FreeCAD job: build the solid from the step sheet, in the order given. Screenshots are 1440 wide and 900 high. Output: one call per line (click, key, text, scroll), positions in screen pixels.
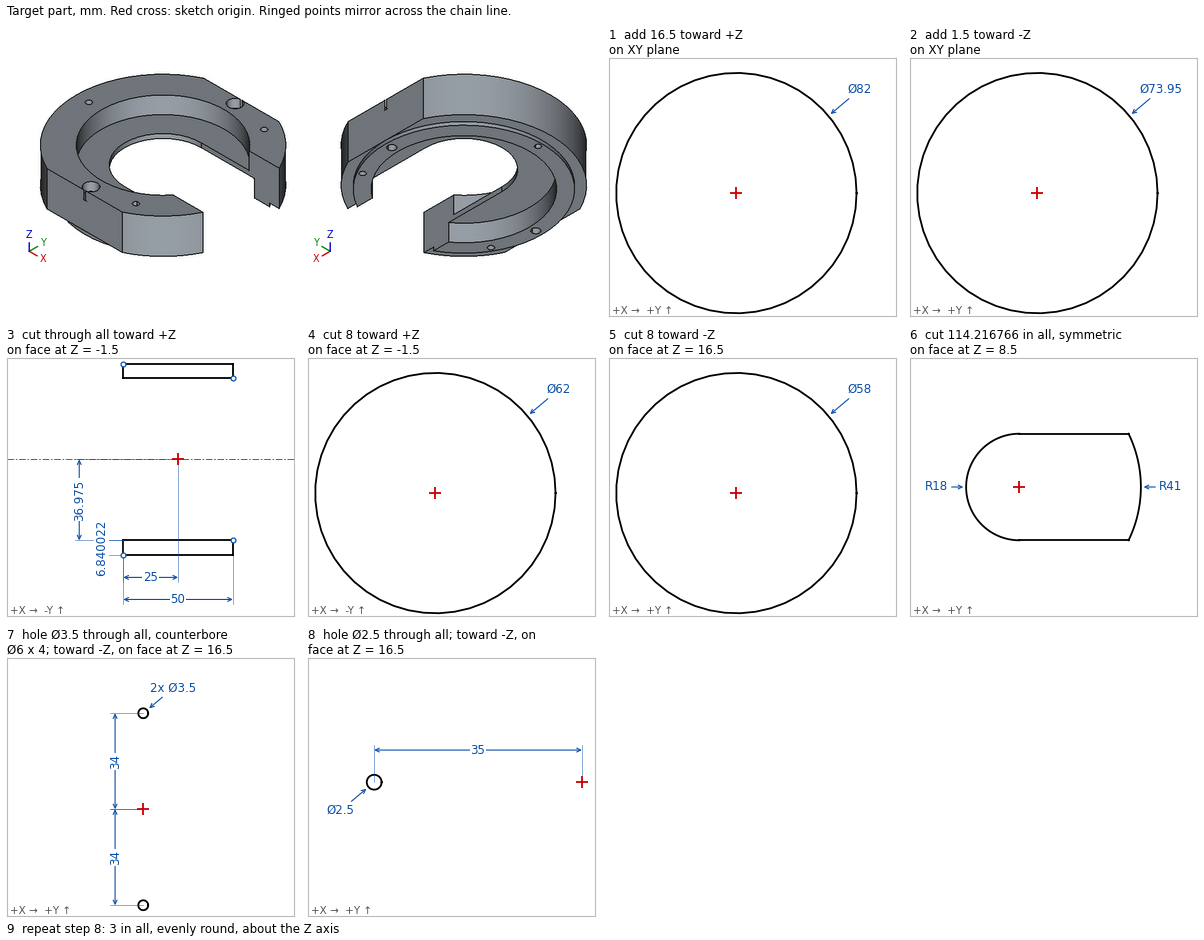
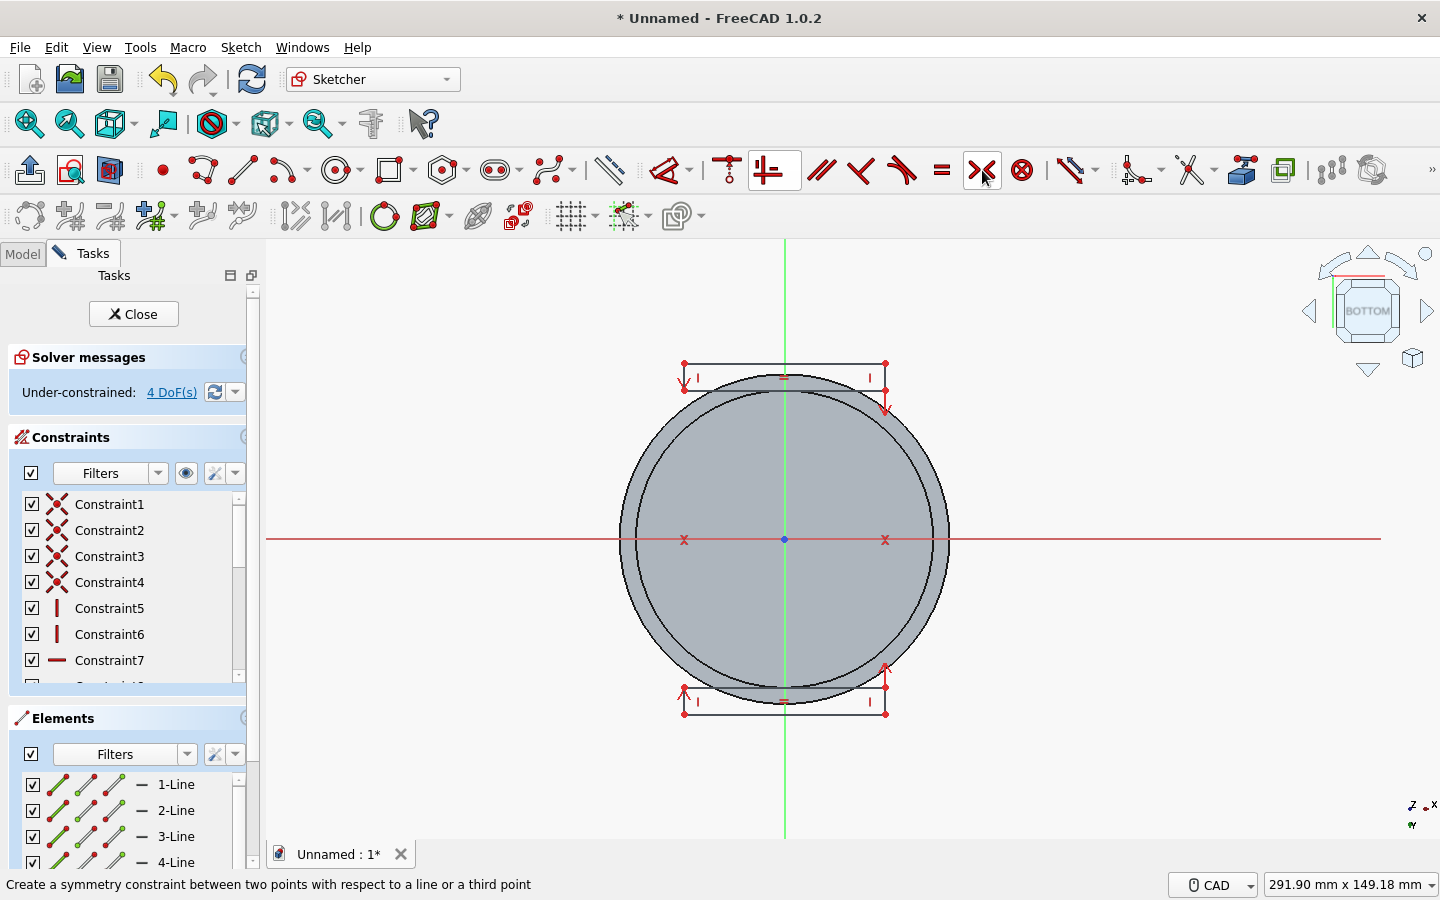
click(664, 170)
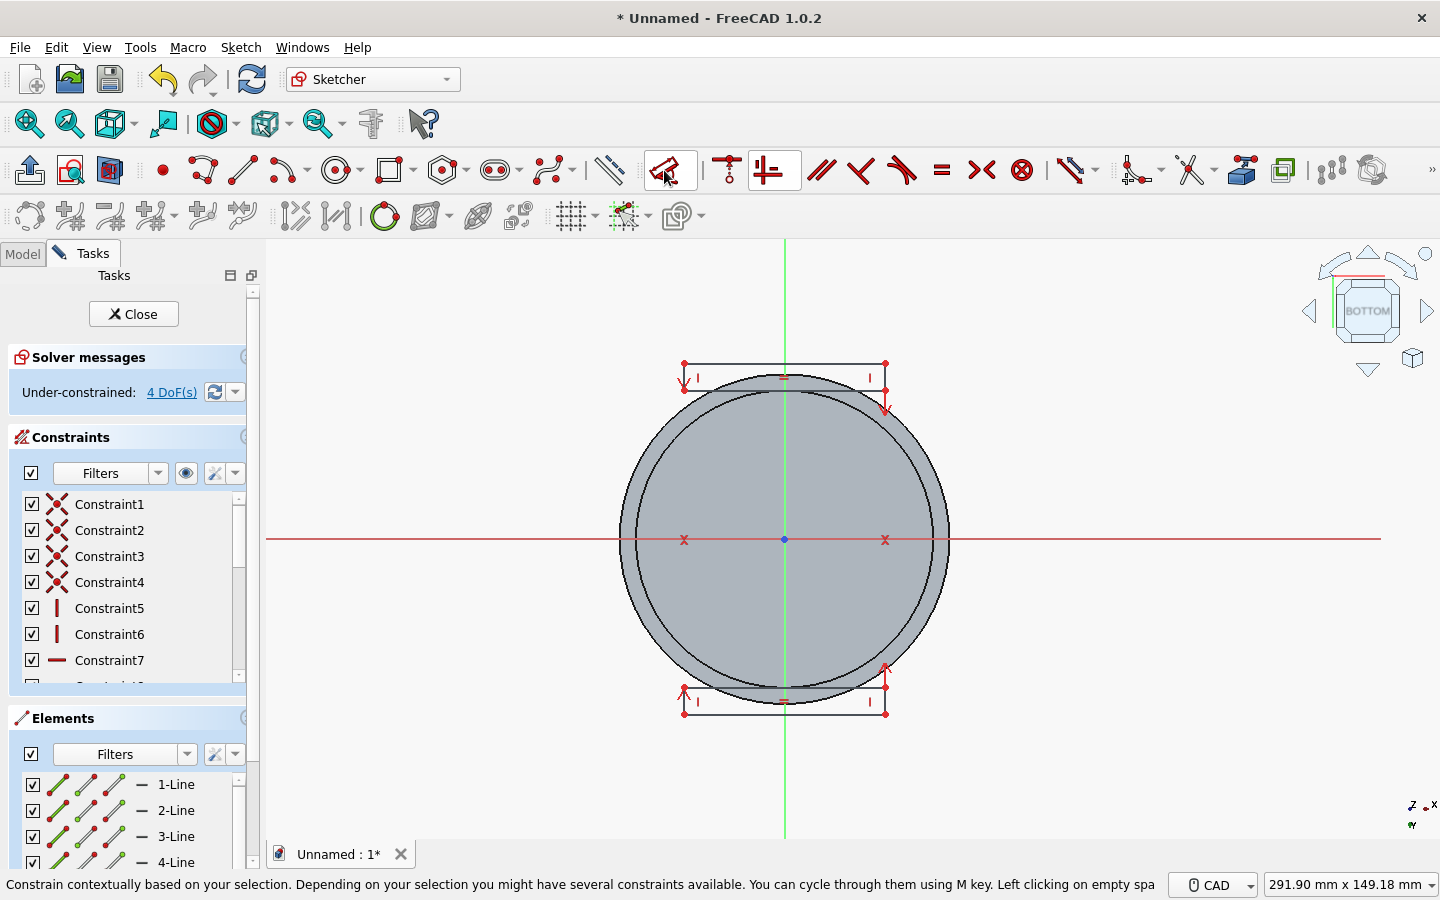
click(744, 715)
click(738, 749)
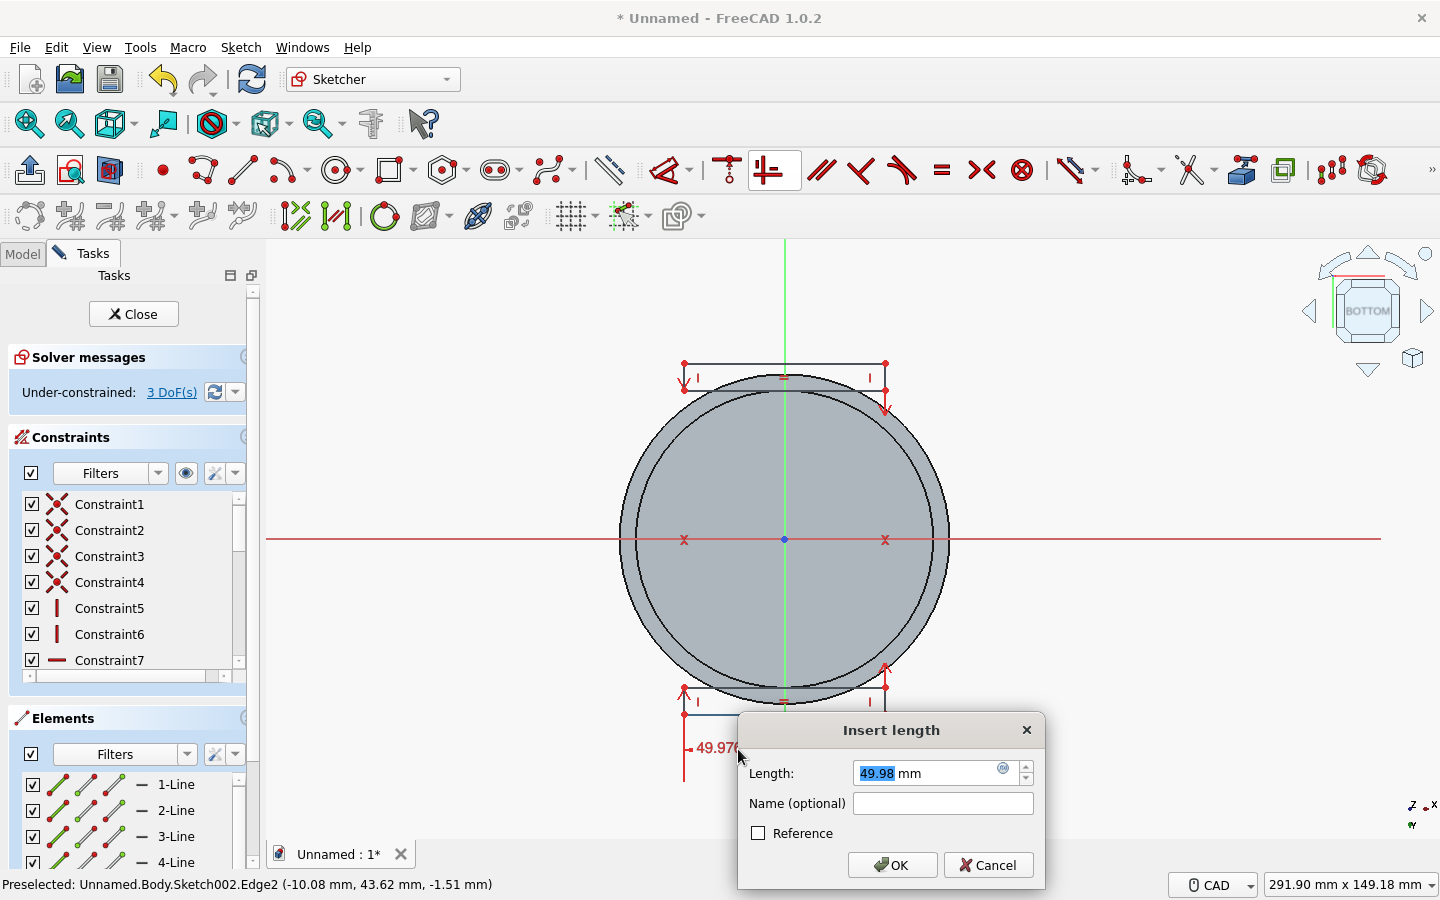
text(50)
key(Return)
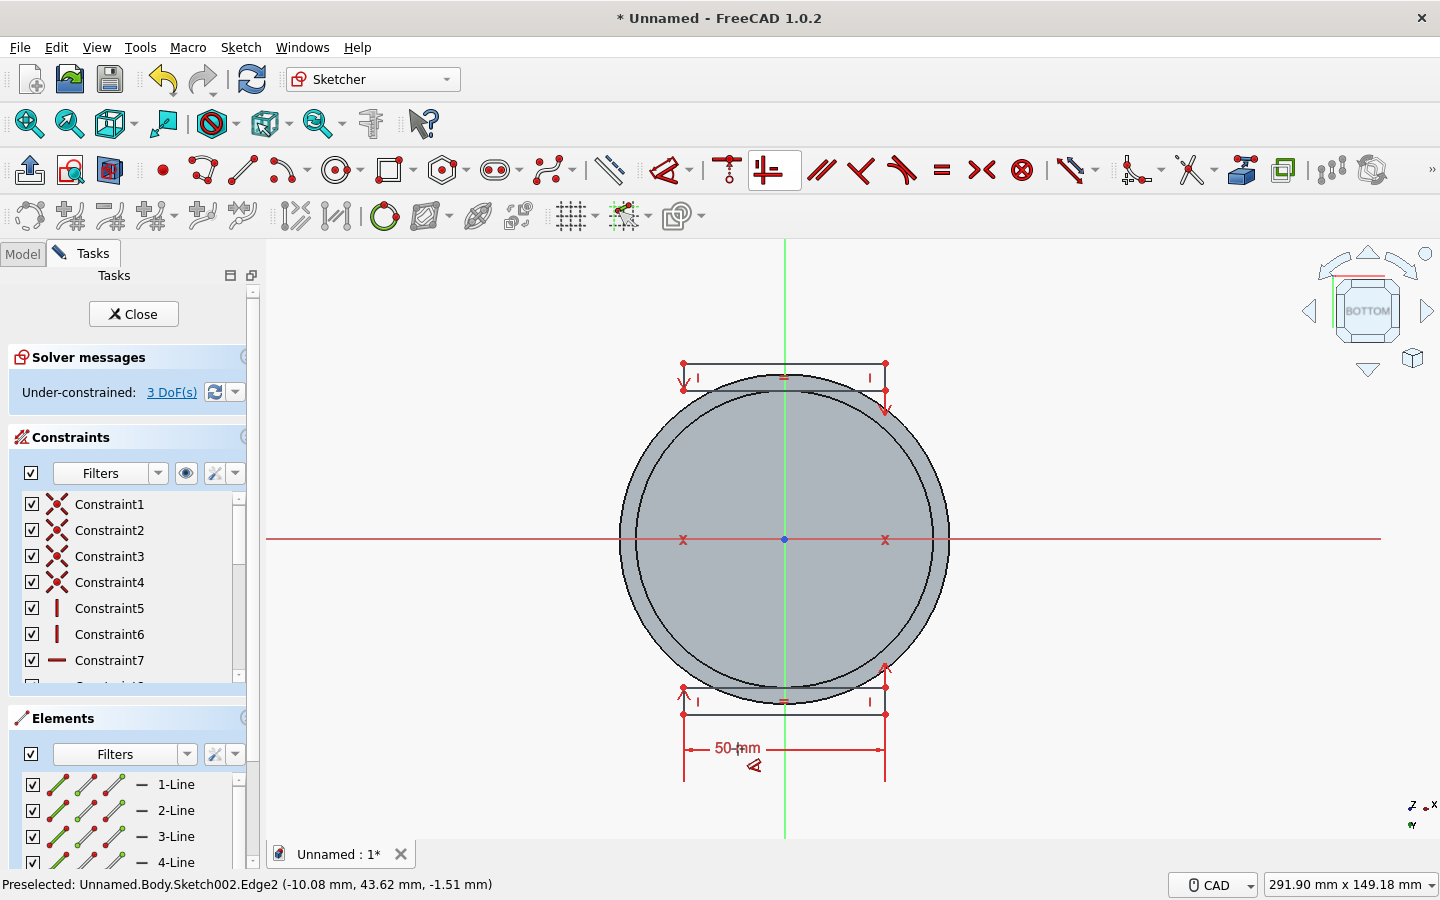
click(684, 688)
click(734, 505)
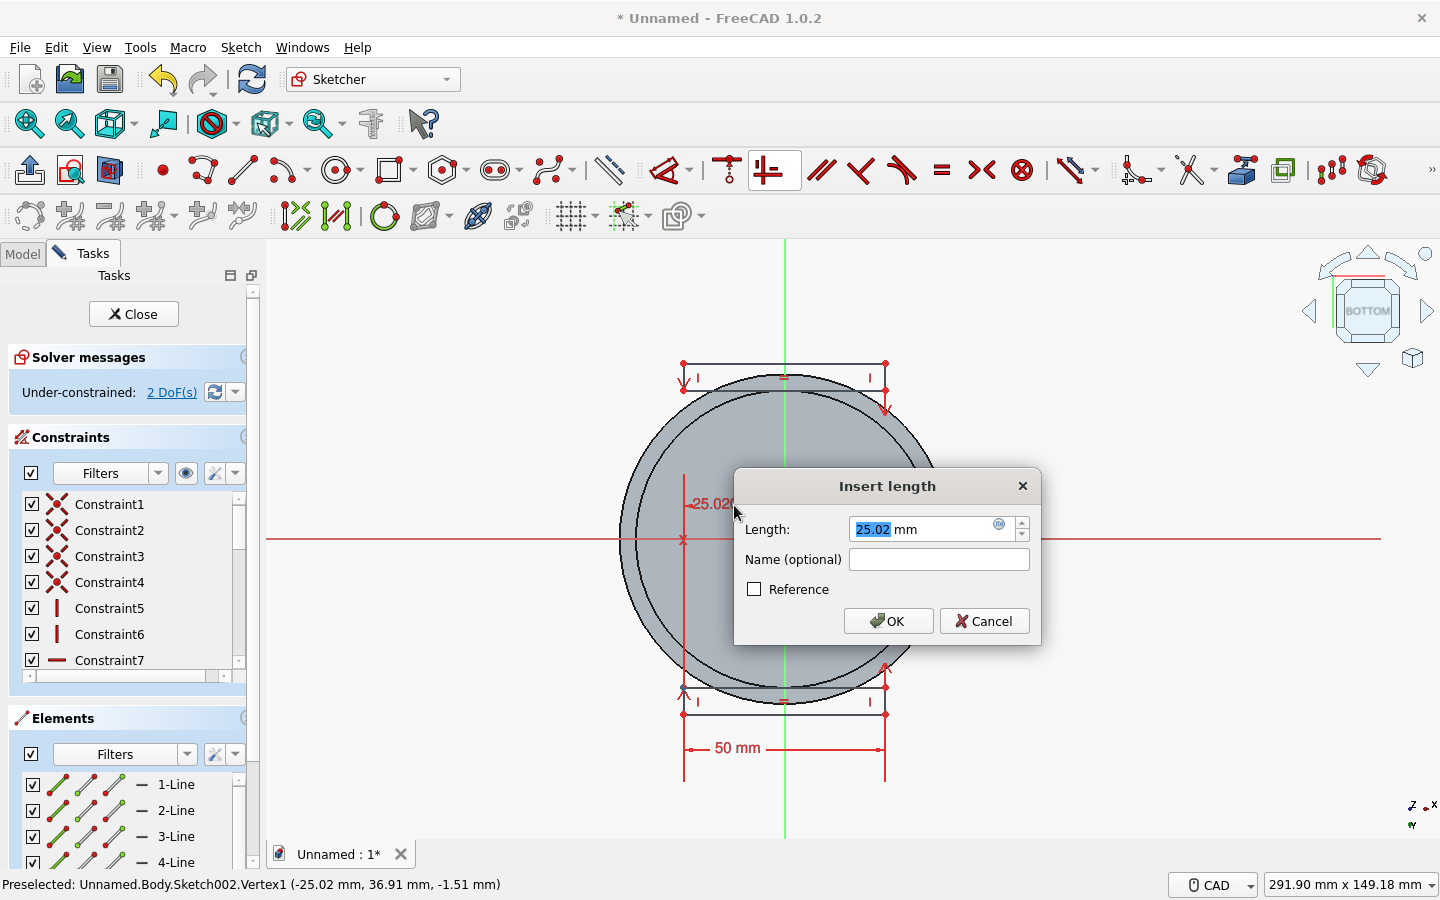
text(25)
key(Return)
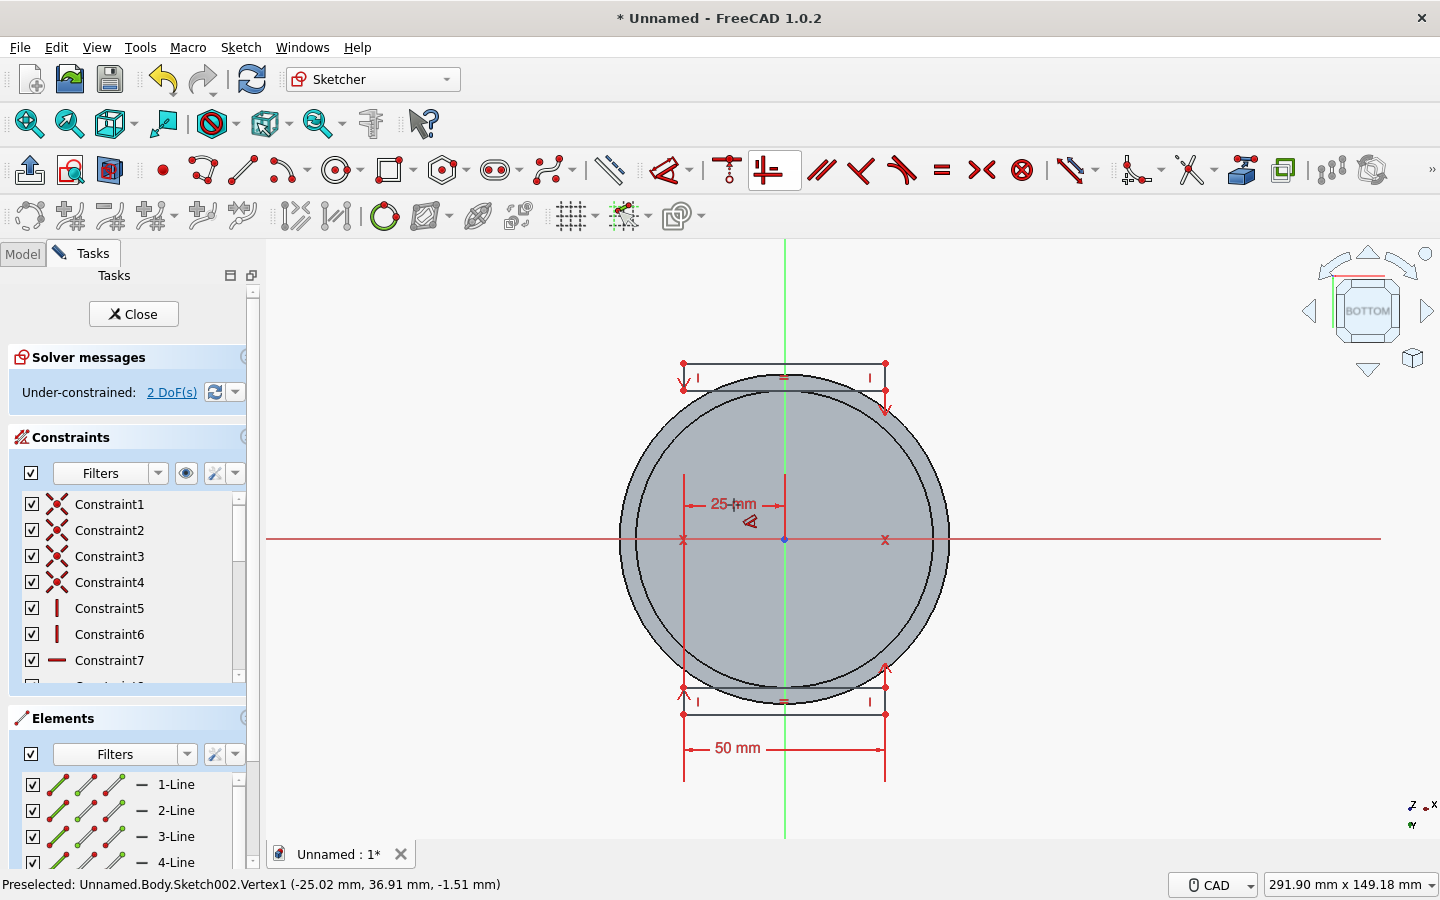
click(684, 688)
click(650, 613)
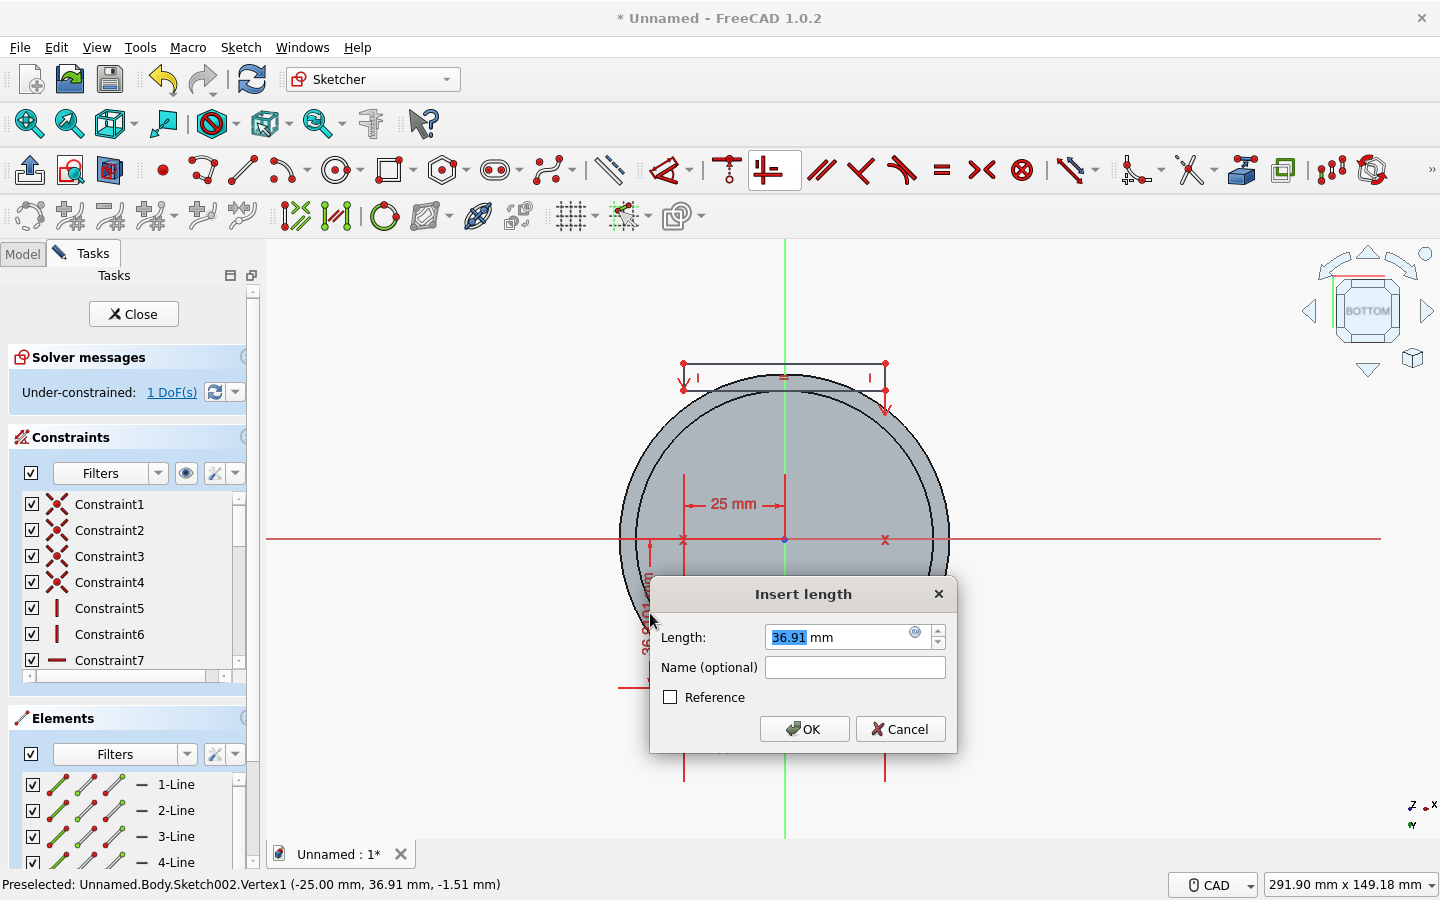
text(36.975)
key(Return)